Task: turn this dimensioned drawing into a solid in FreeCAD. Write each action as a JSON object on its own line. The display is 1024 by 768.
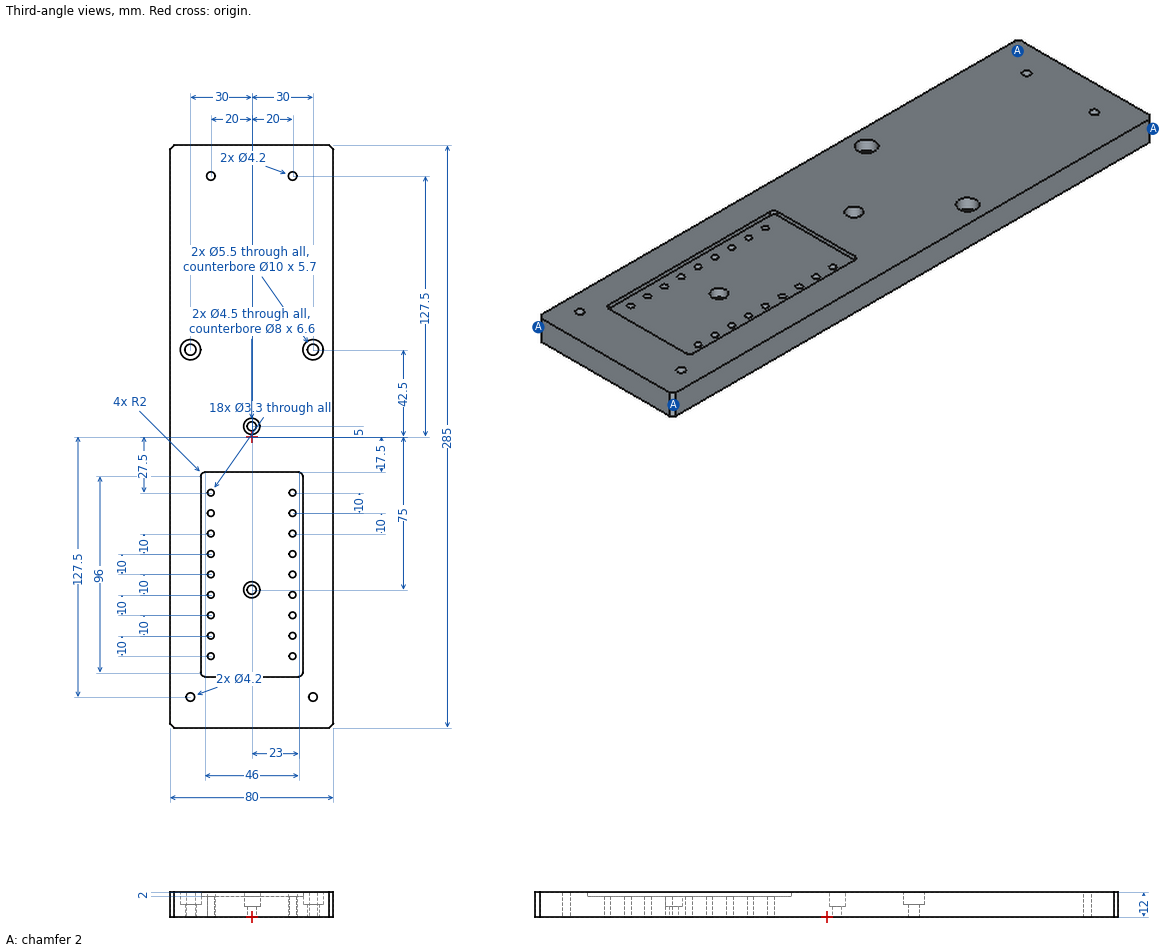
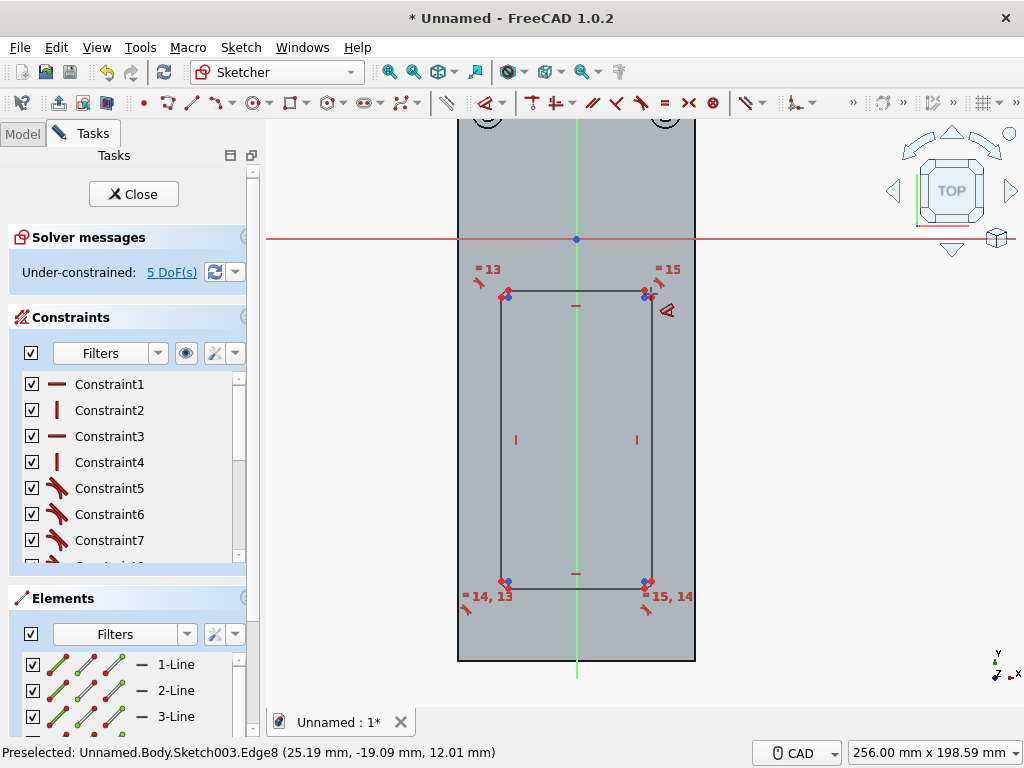
{"action": "scroll", "coordinate": [505, 291], "scroll_direction": "up", "scroll_amount": 10}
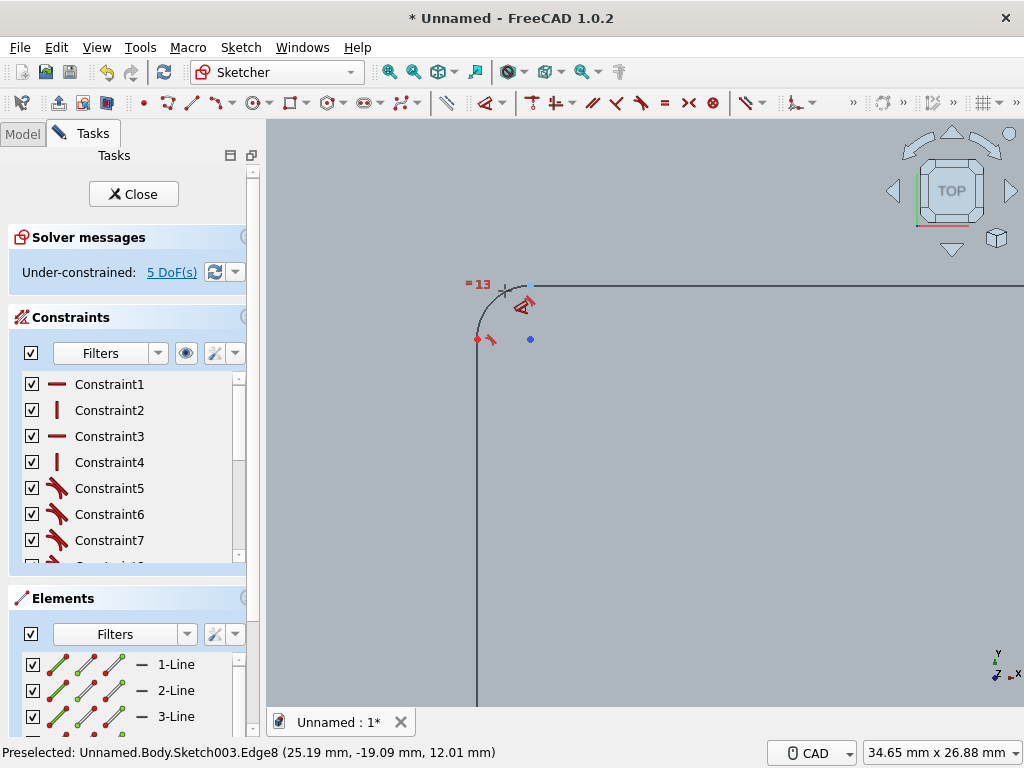
{"action": "left_click", "coordinate": [506, 291]}
{"action": "left_click", "coordinate": [491, 263]}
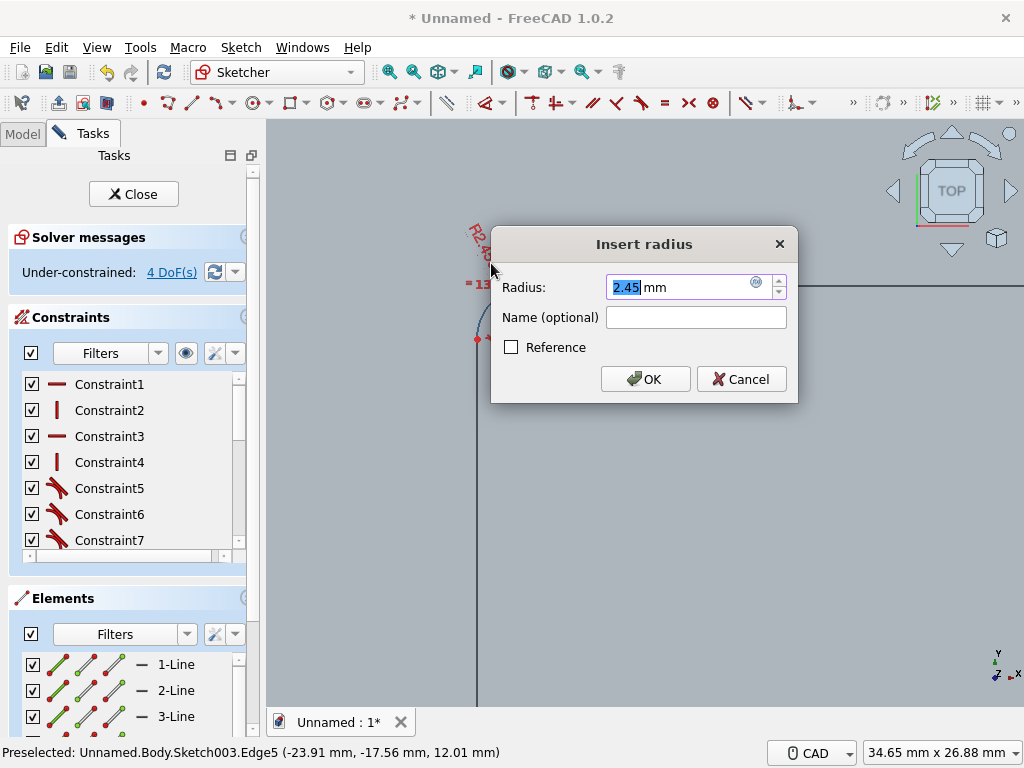
{"action": "type", "text": "2"}
{"action": "key", "text": "Return"}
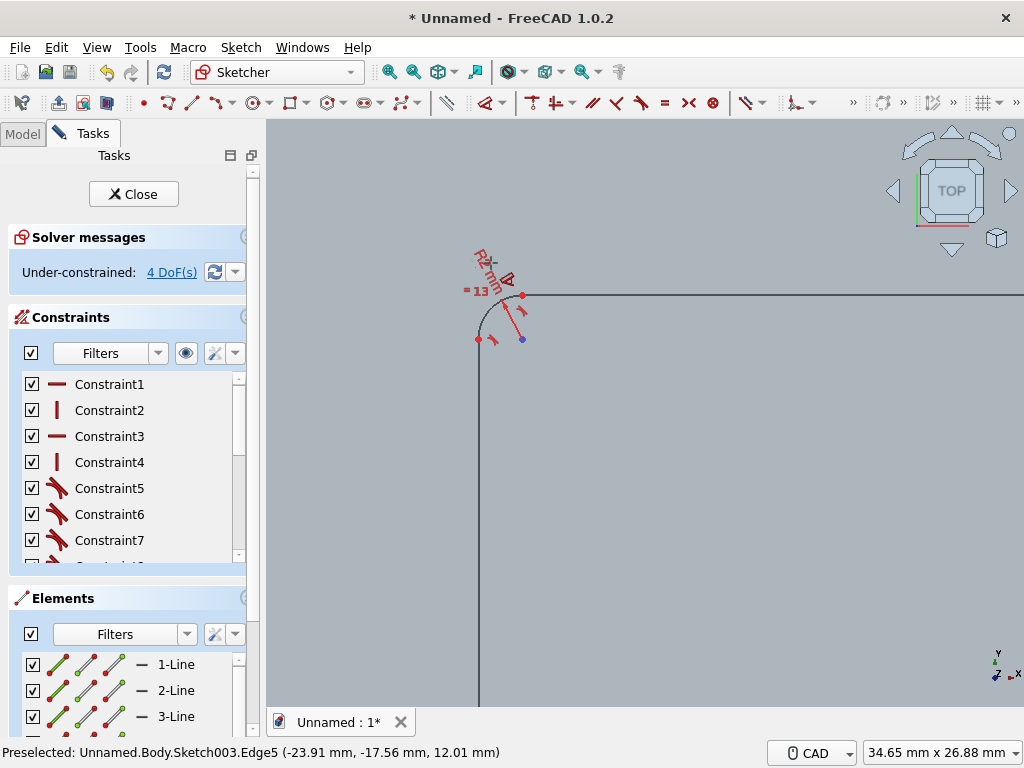
{"action": "scroll", "coordinate": [505, 291], "scroll_direction": "down", "scroll_amount": 10}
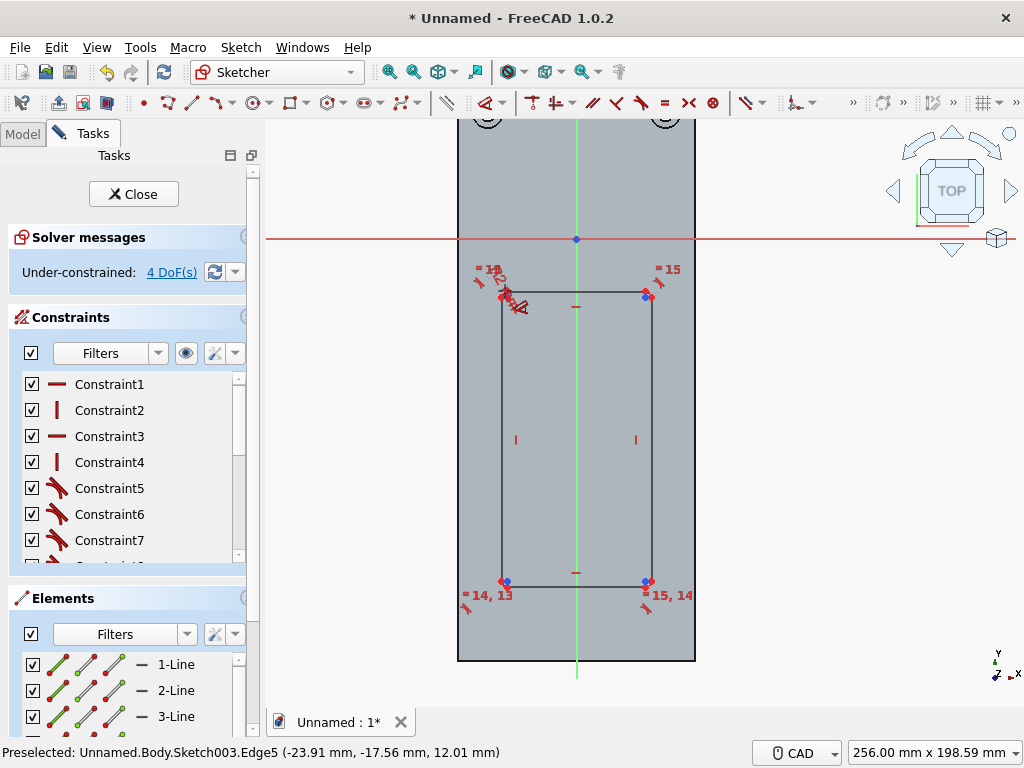
{"action": "left_click", "coordinate": [549, 292]}
{"action": "left_click", "coordinate": [545, 258]}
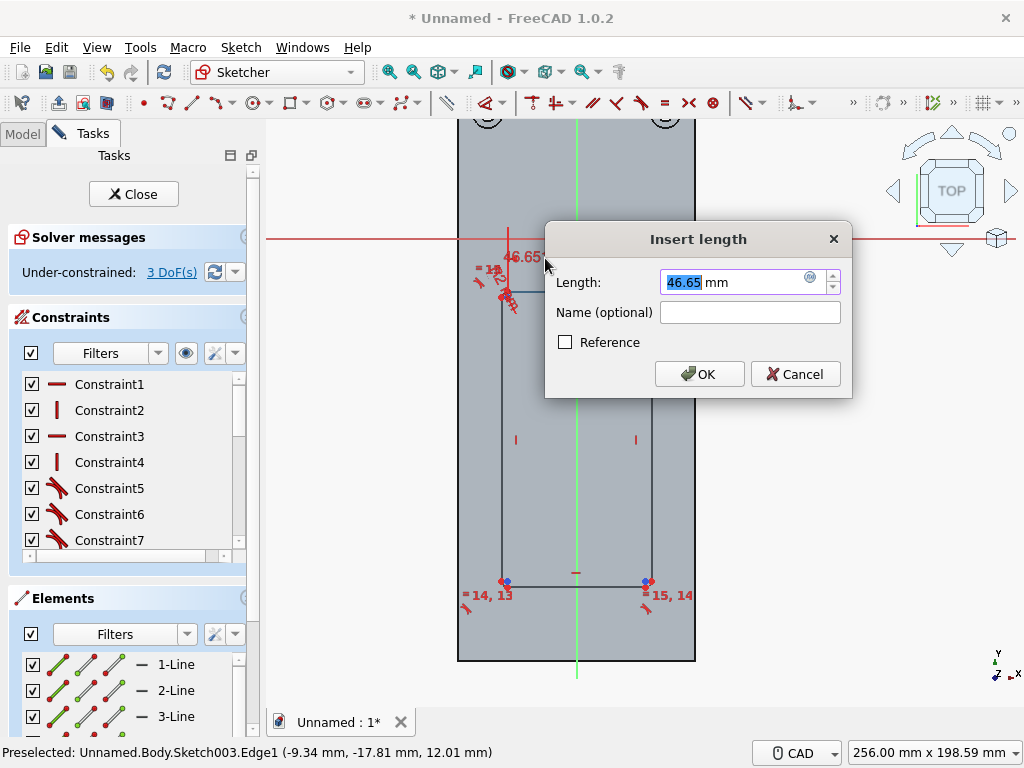
{"action": "type", "text": "46"}
{"action": "key", "text": "Return"}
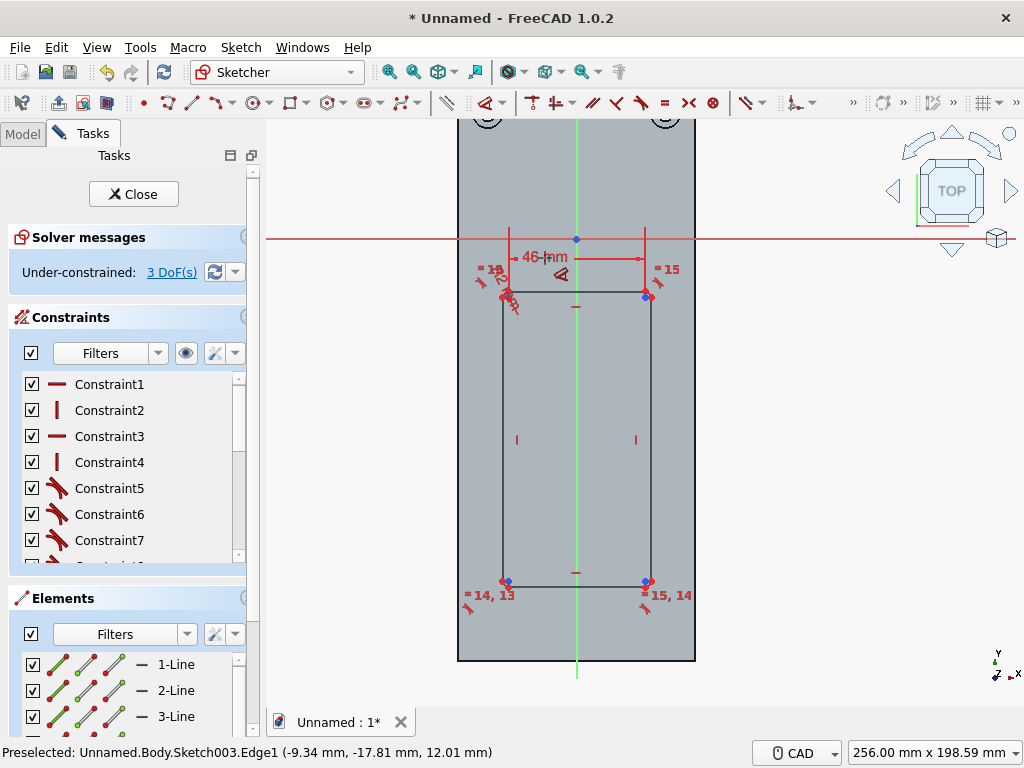
{"action": "left_click", "coordinate": [503, 383]}
{"action": "left_click", "coordinate": [469, 440]}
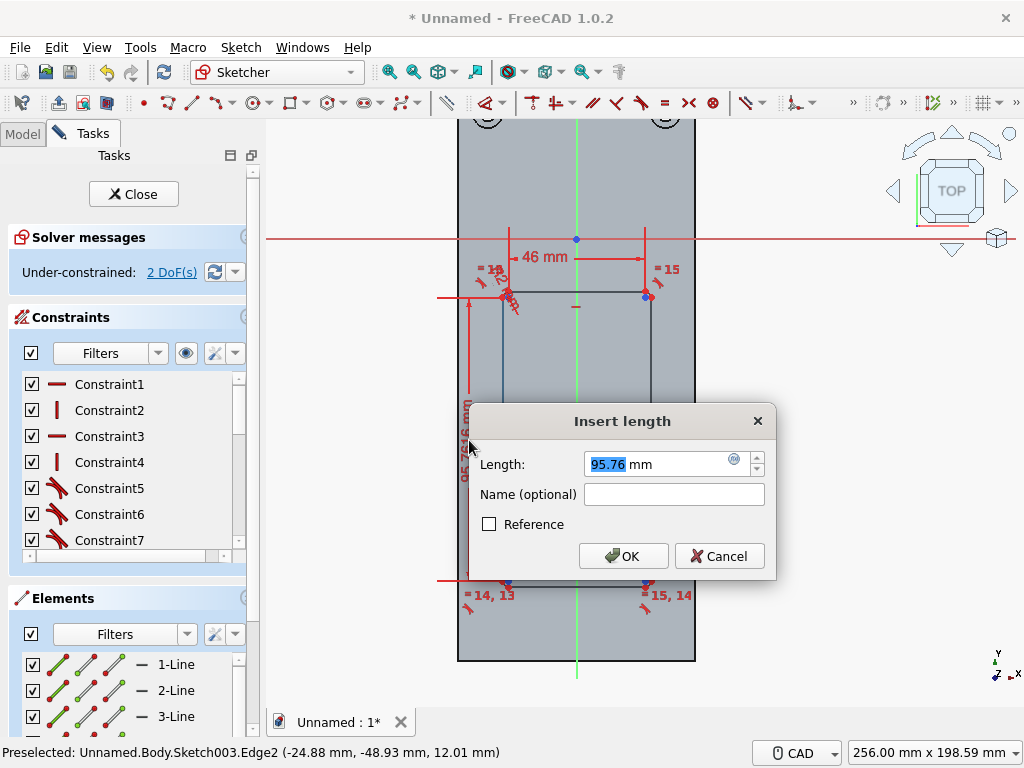
{"action": "type", "text": "96"}
{"action": "key", "text": "Return"}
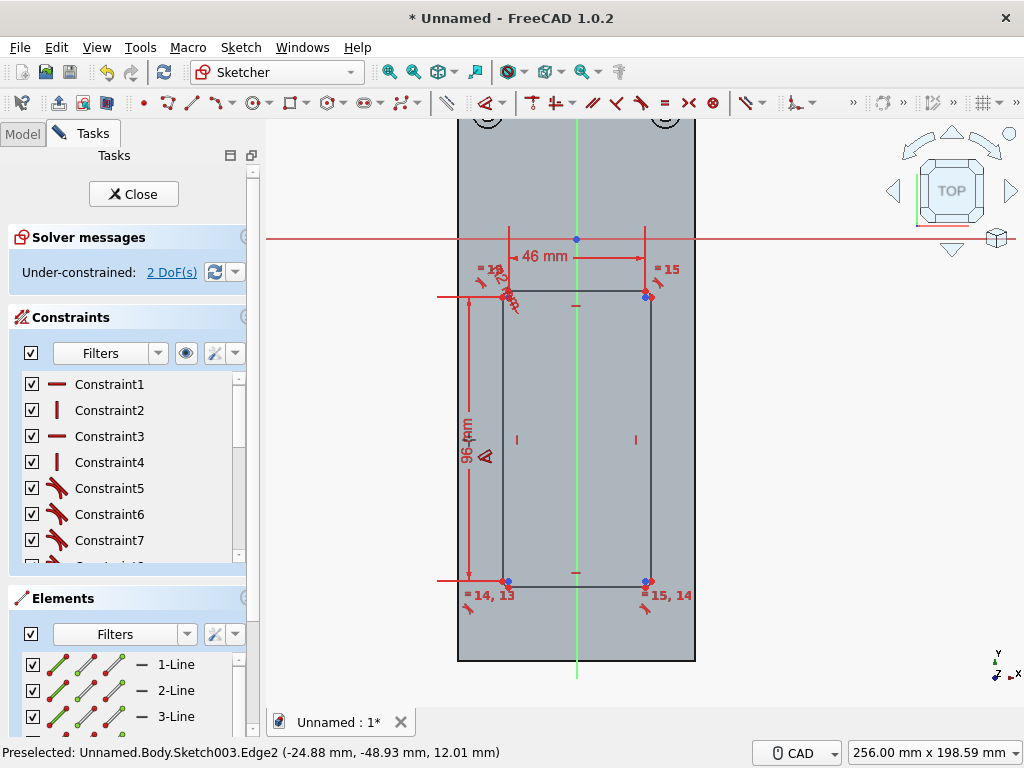
{"action": "scroll", "coordinate": [645, 291], "scroll_direction": "up", "scroll_amount": 4}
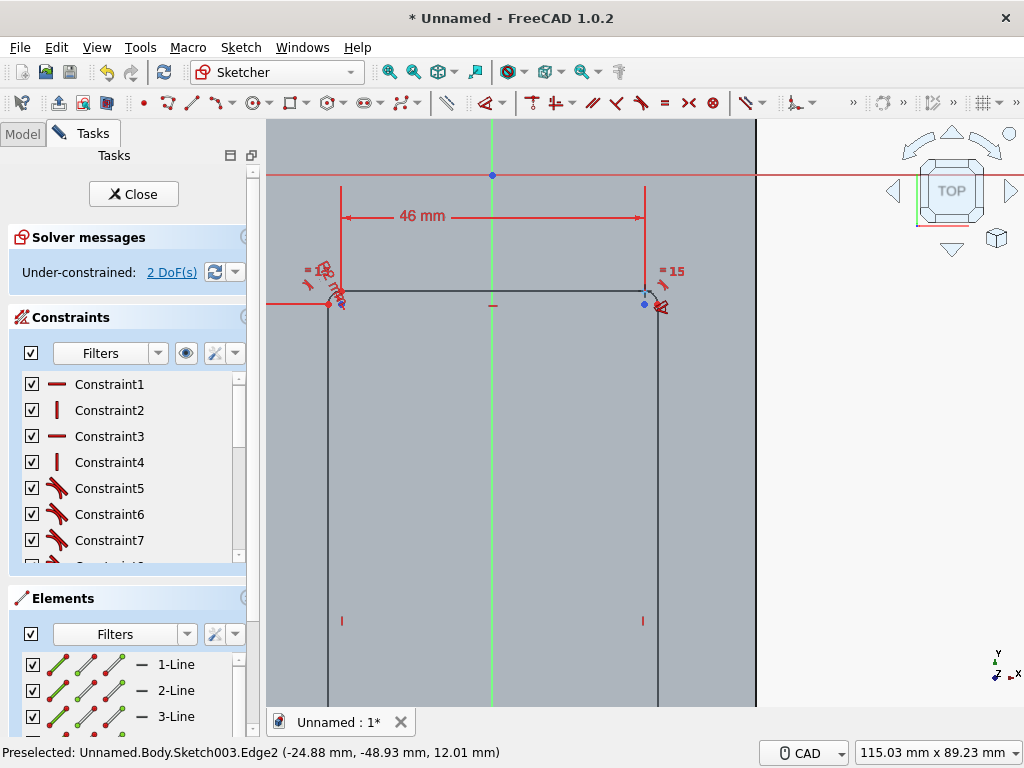
{"action": "left_click", "coordinate": [645, 291]}
{"action": "left_click", "coordinate": [568, 325]}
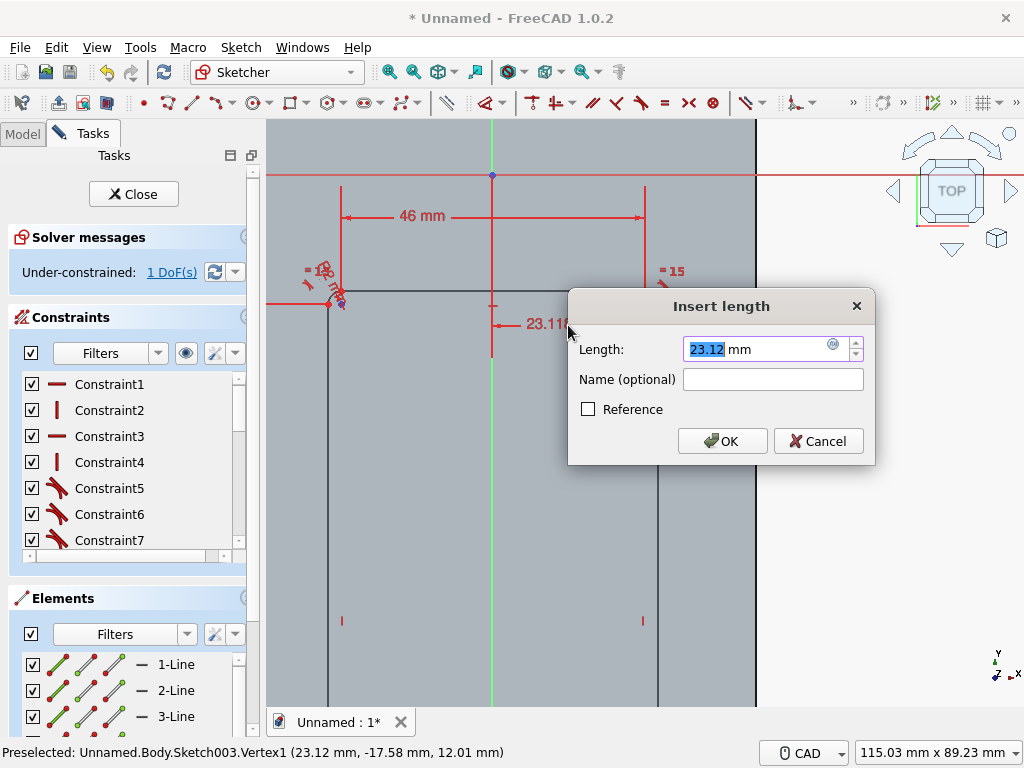
{"action": "type", "text": "23"}
{"action": "key", "text": "Return"}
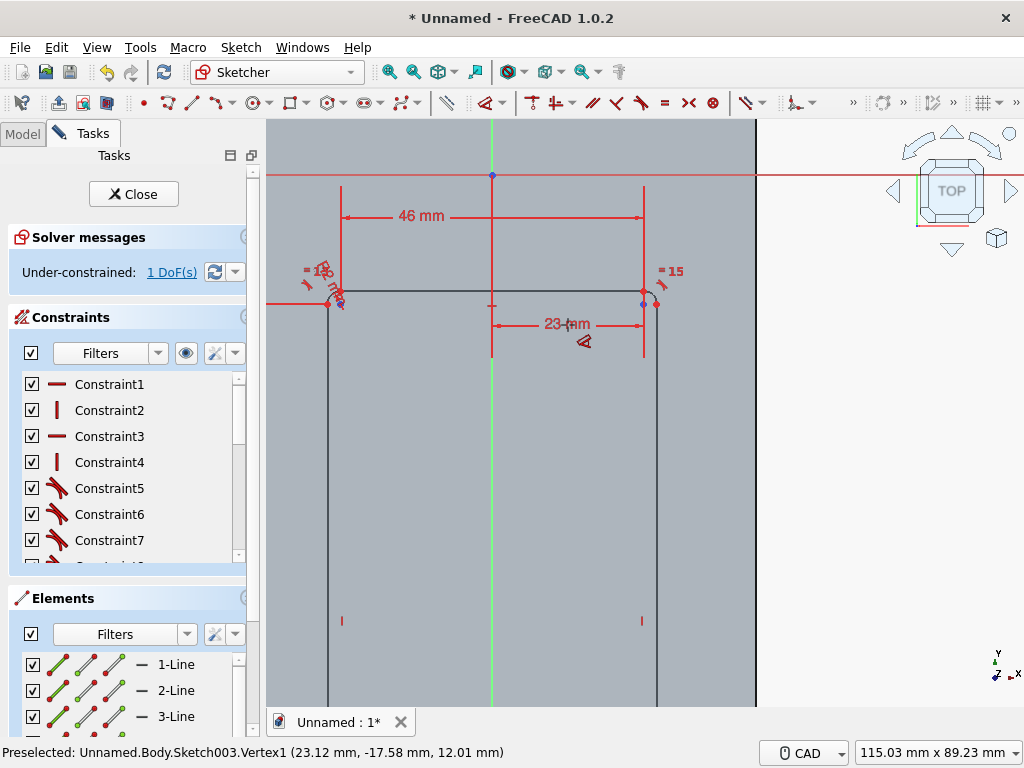
{"action": "left_click", "coordinate": [644, 291]}
{"action": "left_click", "coordinate": [678, 233]}